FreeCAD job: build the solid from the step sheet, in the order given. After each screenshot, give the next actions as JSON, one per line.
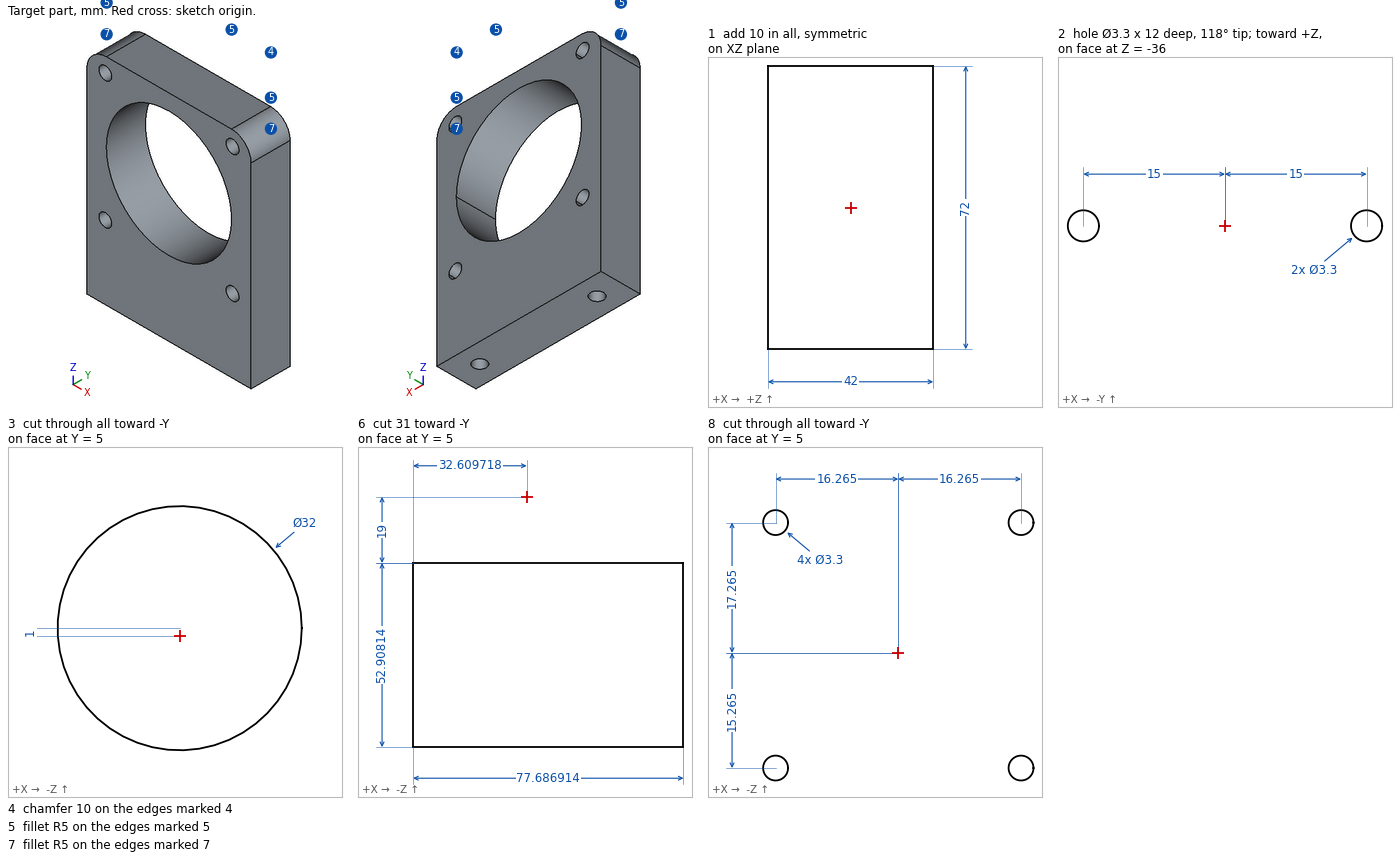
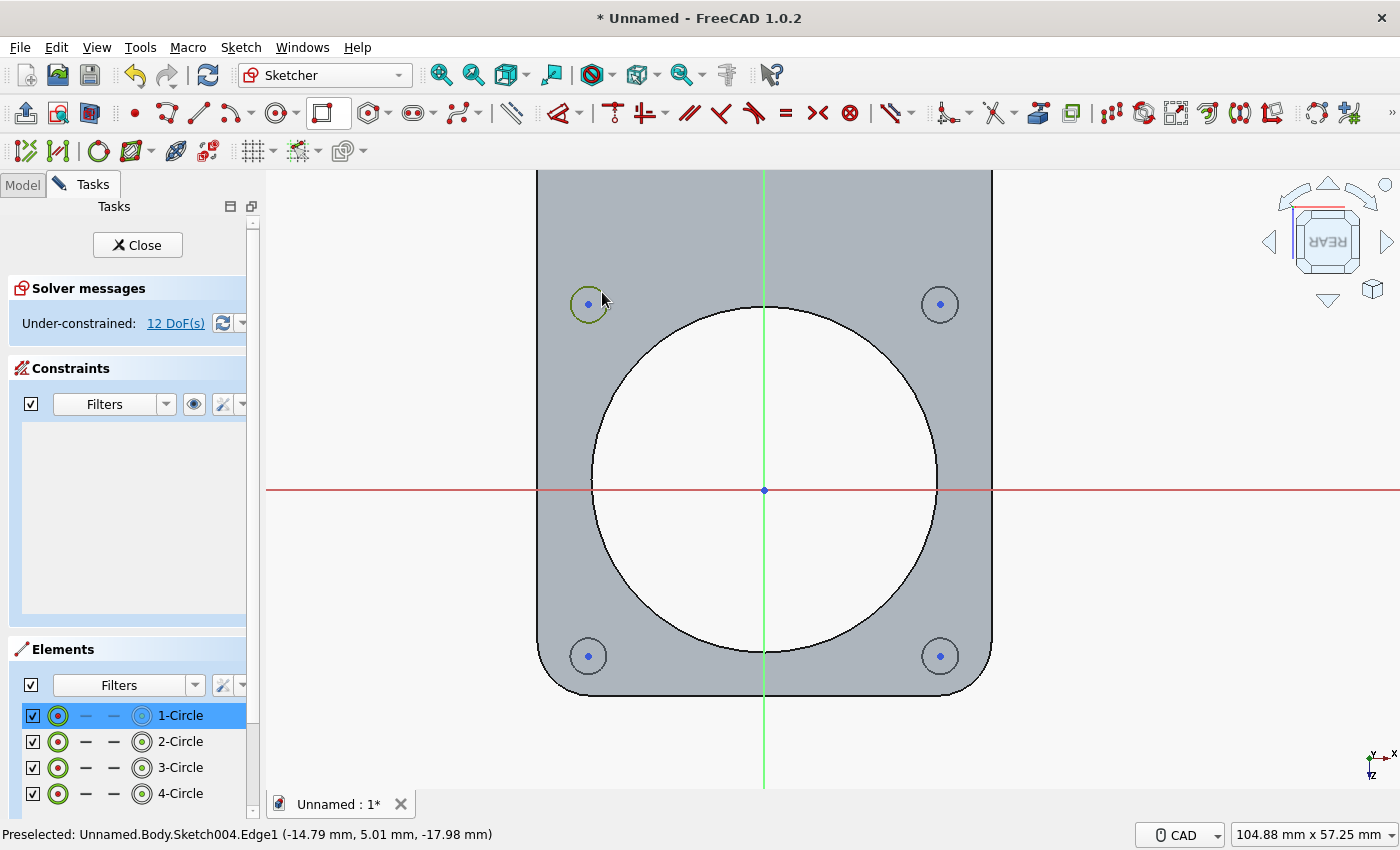
{"action": "left_click", "coordinate": [953, 292]}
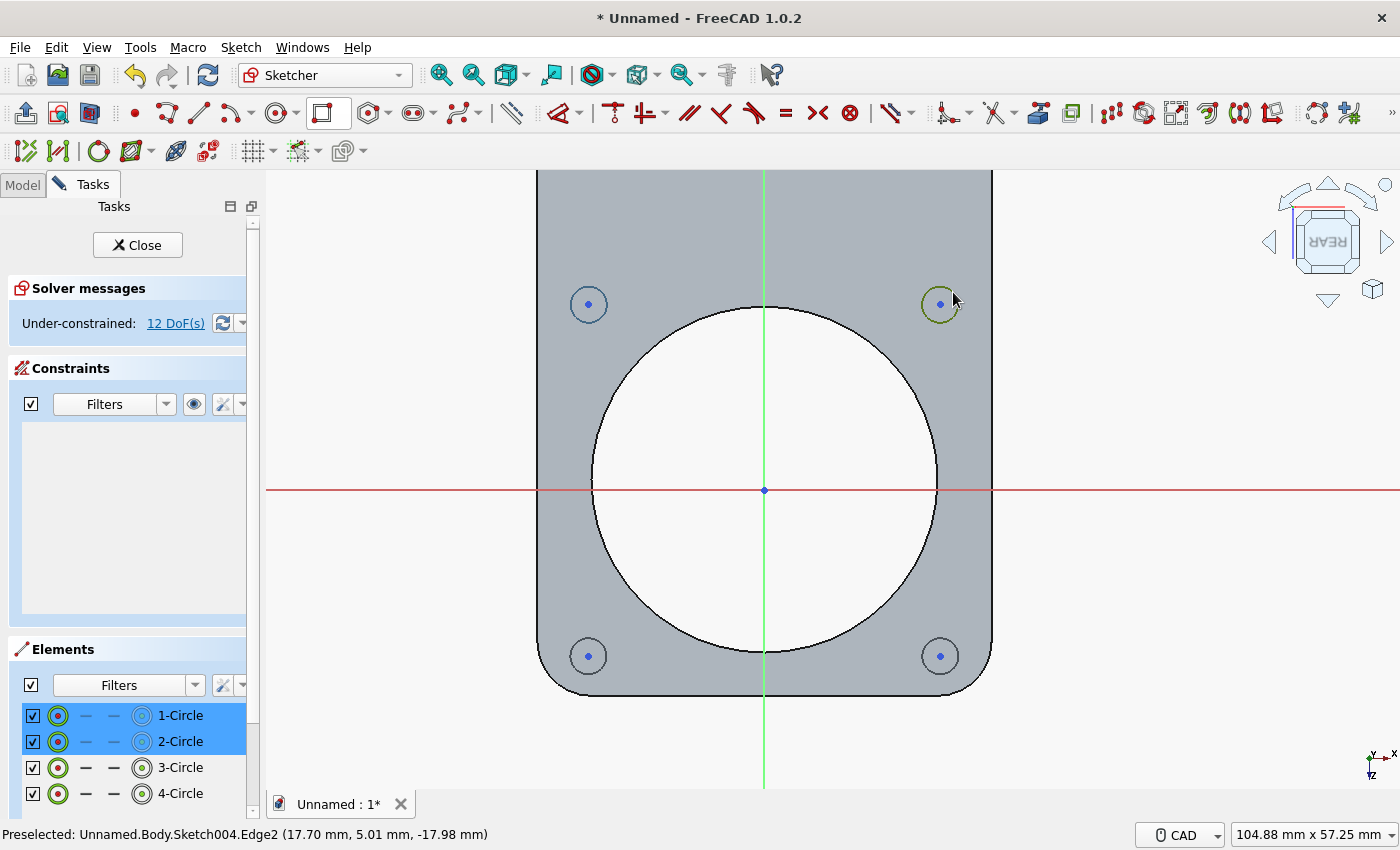
{"action": "left_click", "coordinate": [601, 643]}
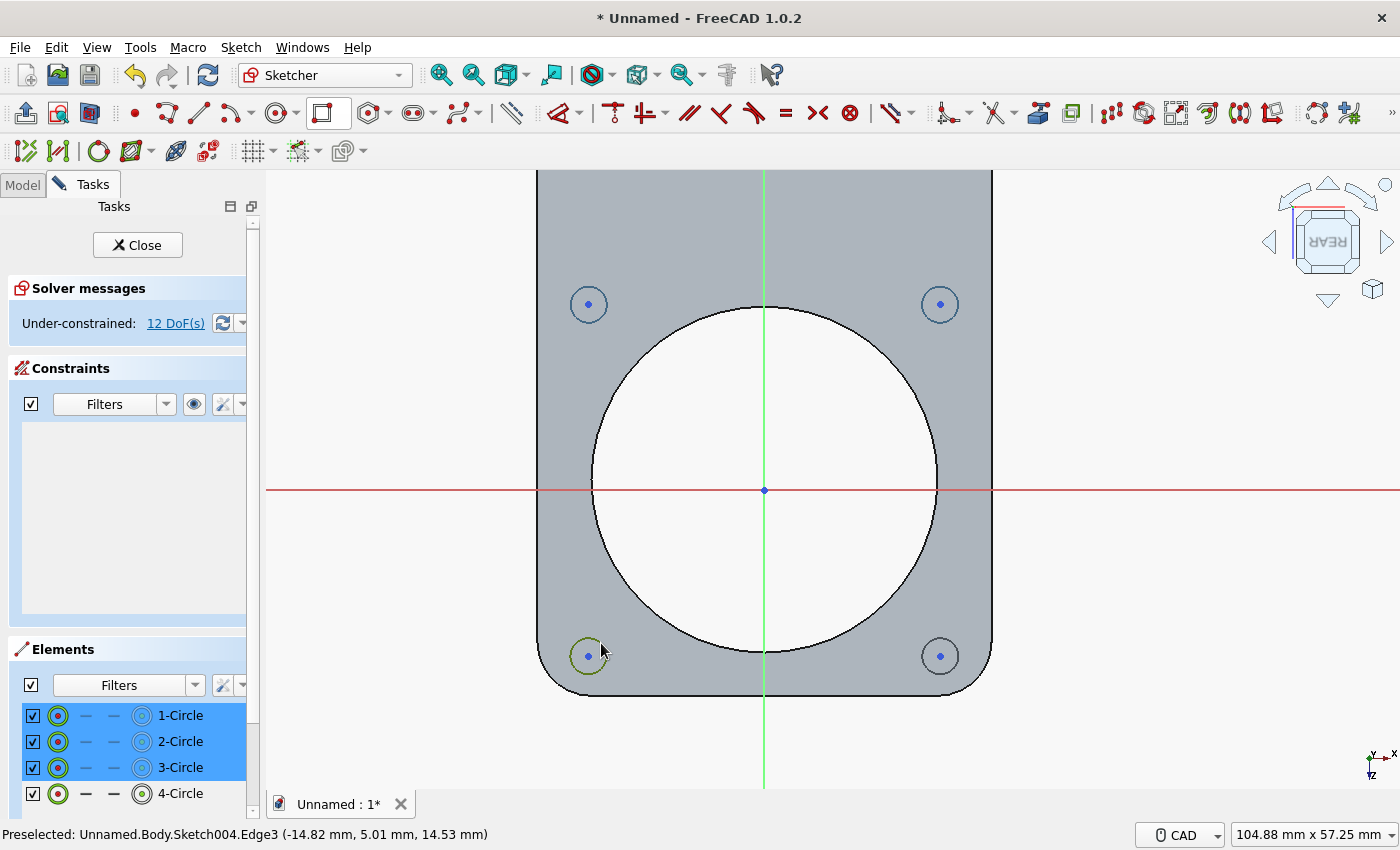
{"action": "left_click", "coordinate": [953, 643]}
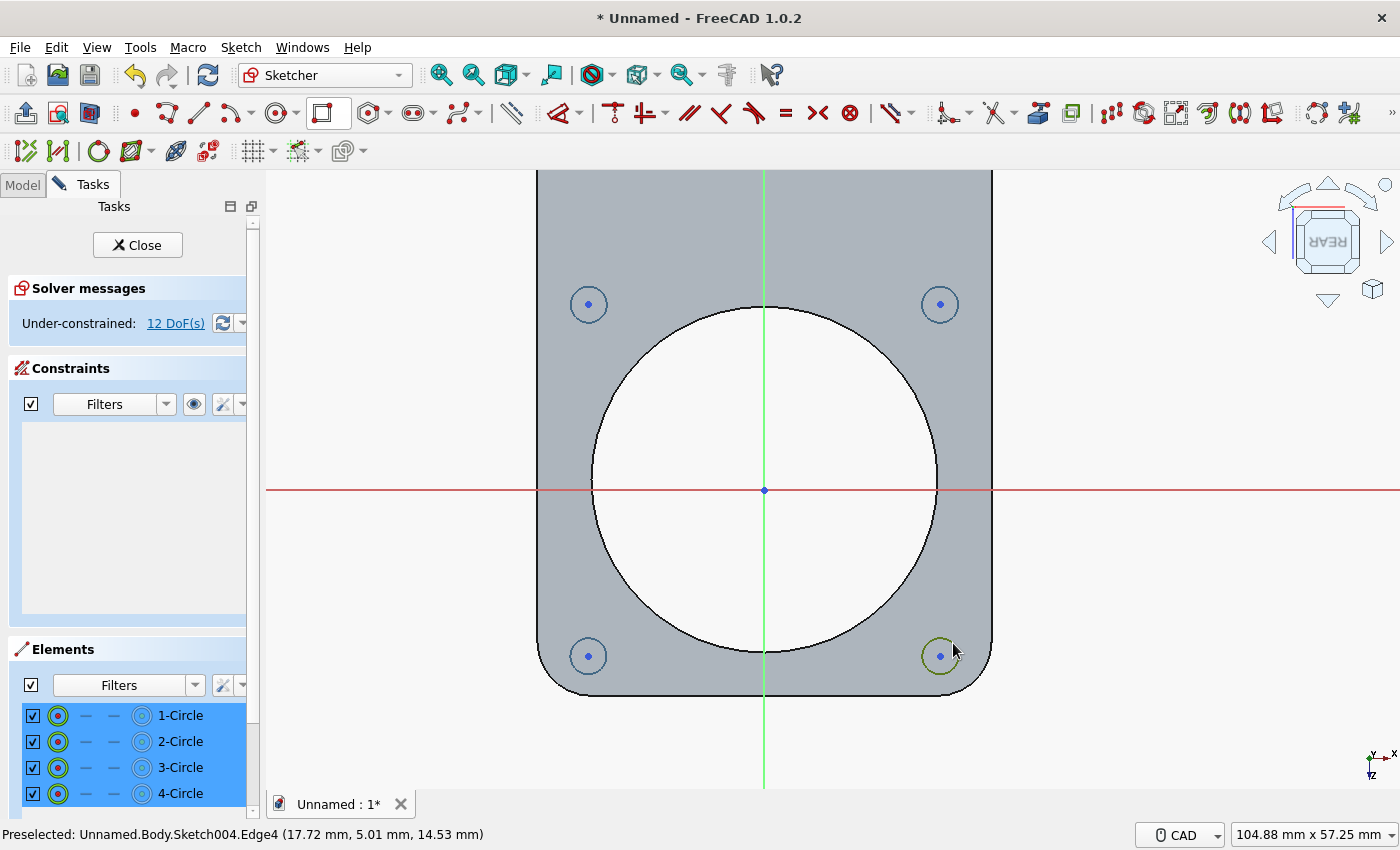
{"action": "left_click", "coordinate": [786, 114]}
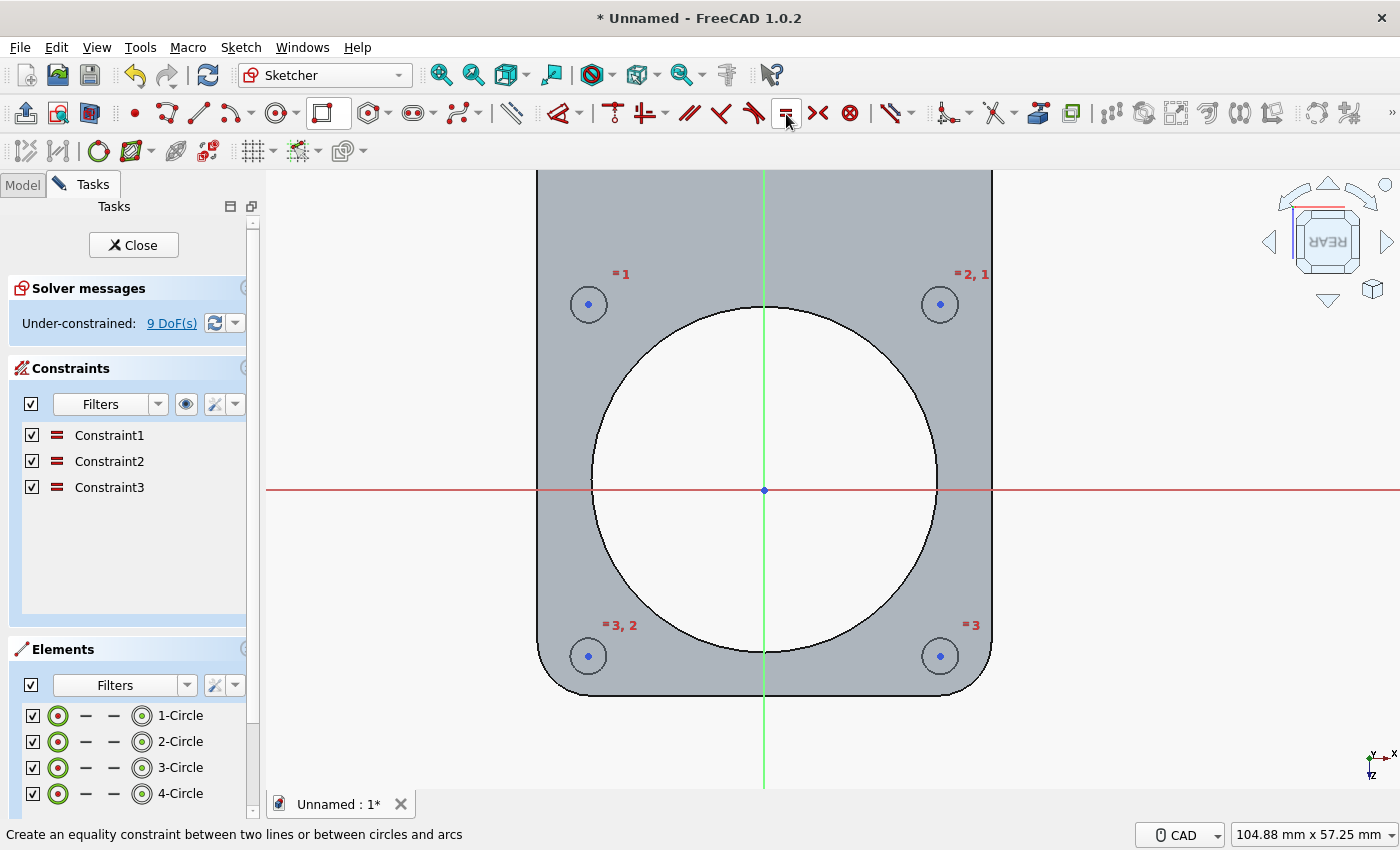
{"action": "left_click", "coordinate": [589, 305]}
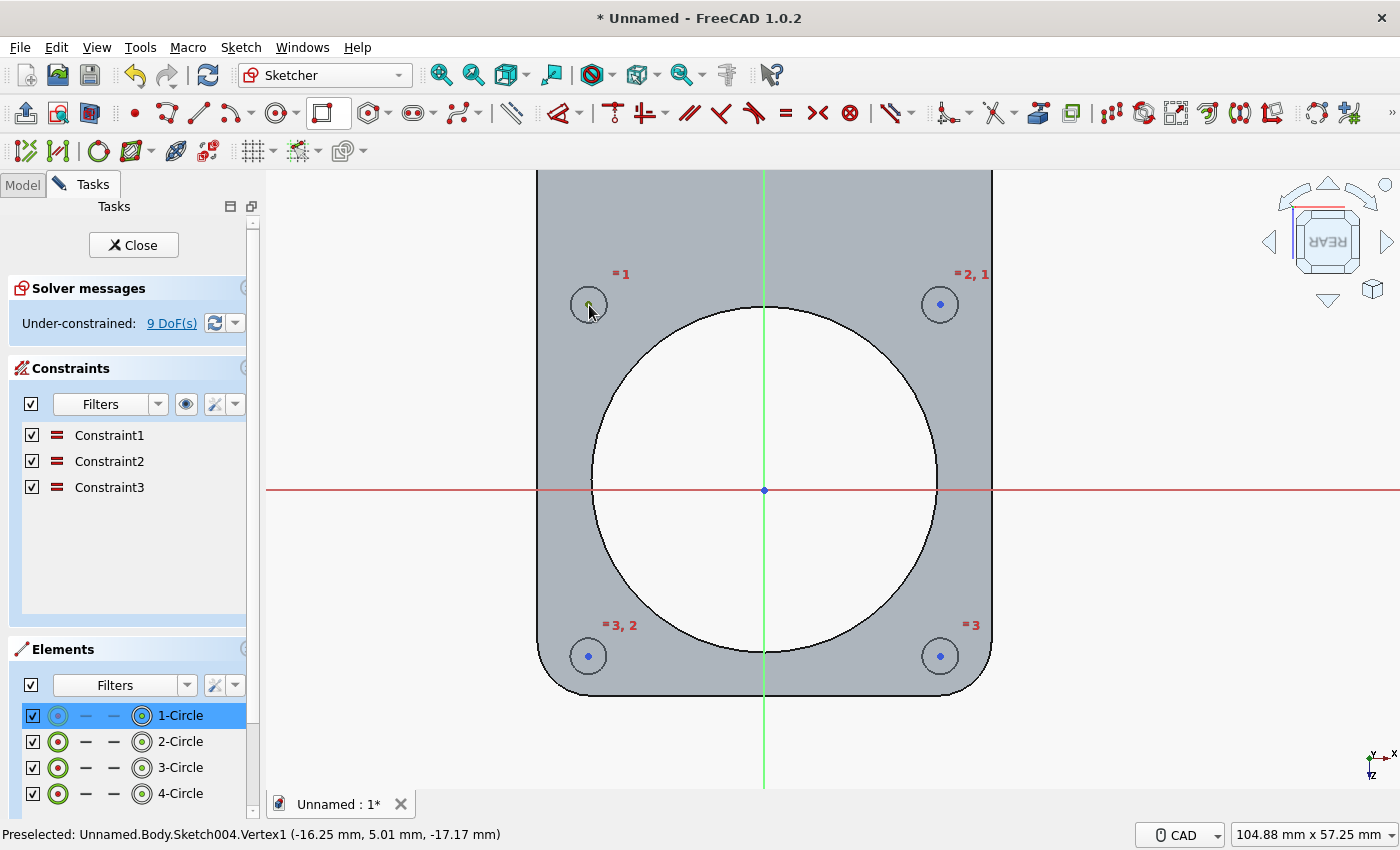
{"action": "left_click", "coordinate": [940, 305]}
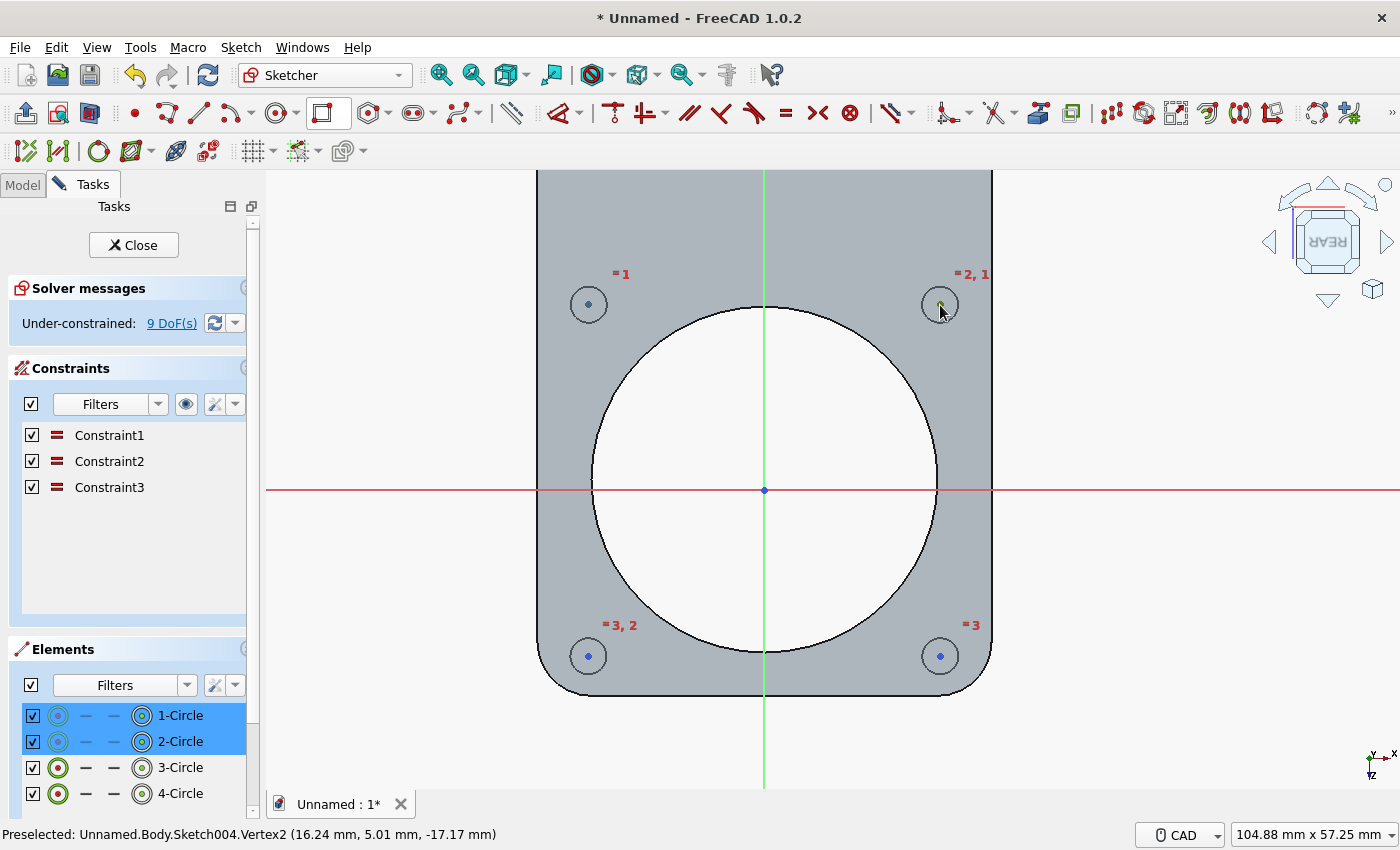
{"action": "left_click", "coordinate": [668, 114]}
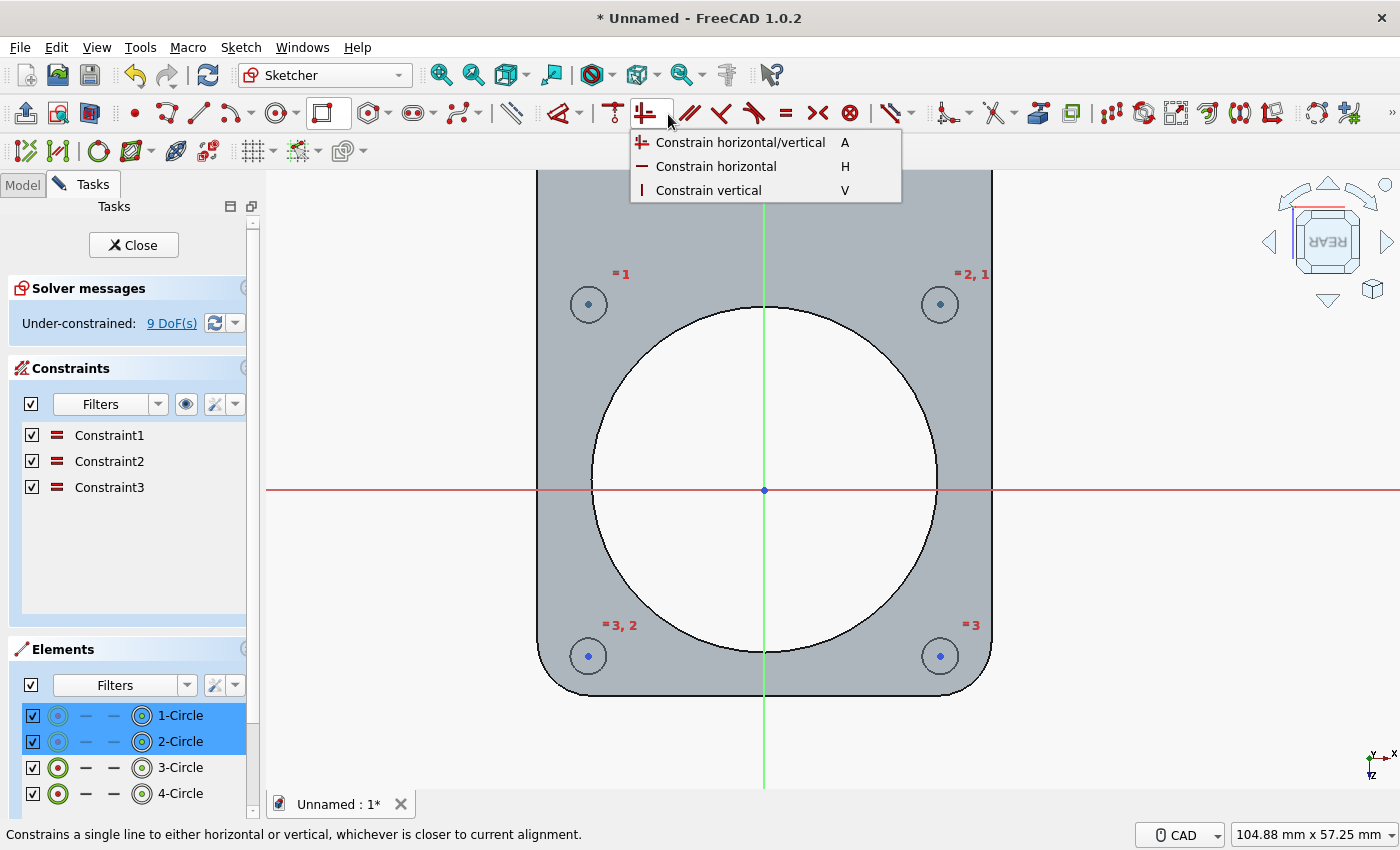
{"action": "left_click", "coordinate": [766, 166]}